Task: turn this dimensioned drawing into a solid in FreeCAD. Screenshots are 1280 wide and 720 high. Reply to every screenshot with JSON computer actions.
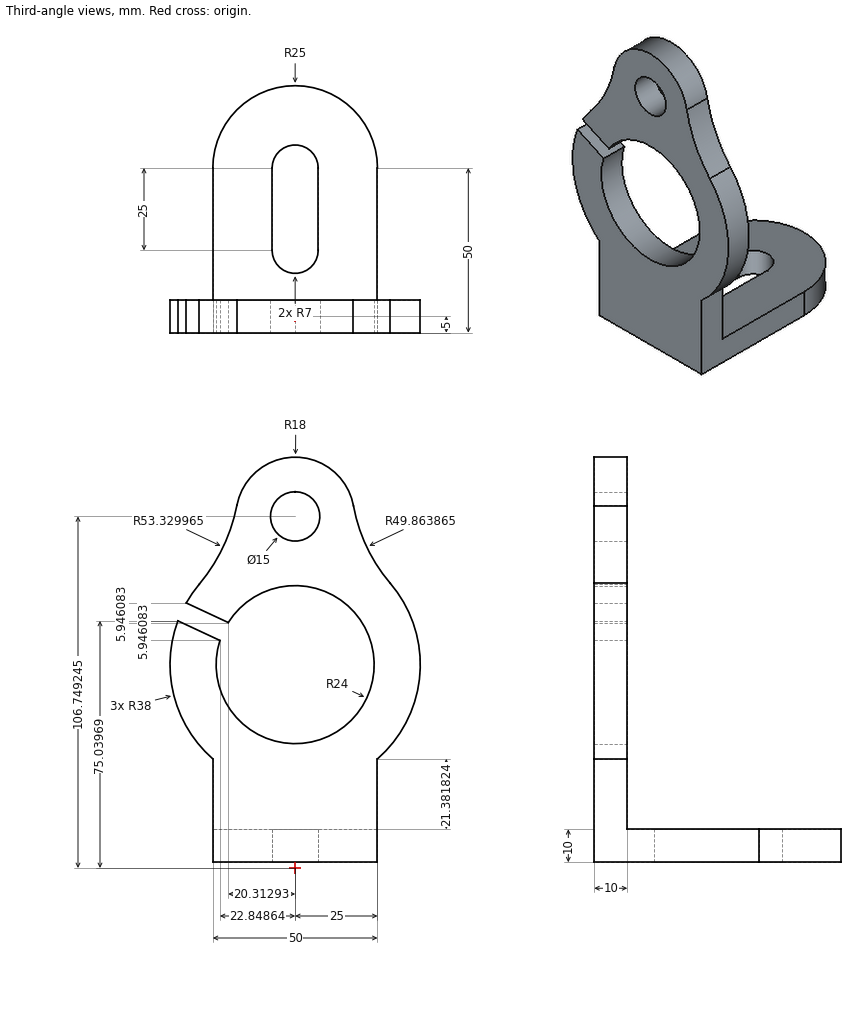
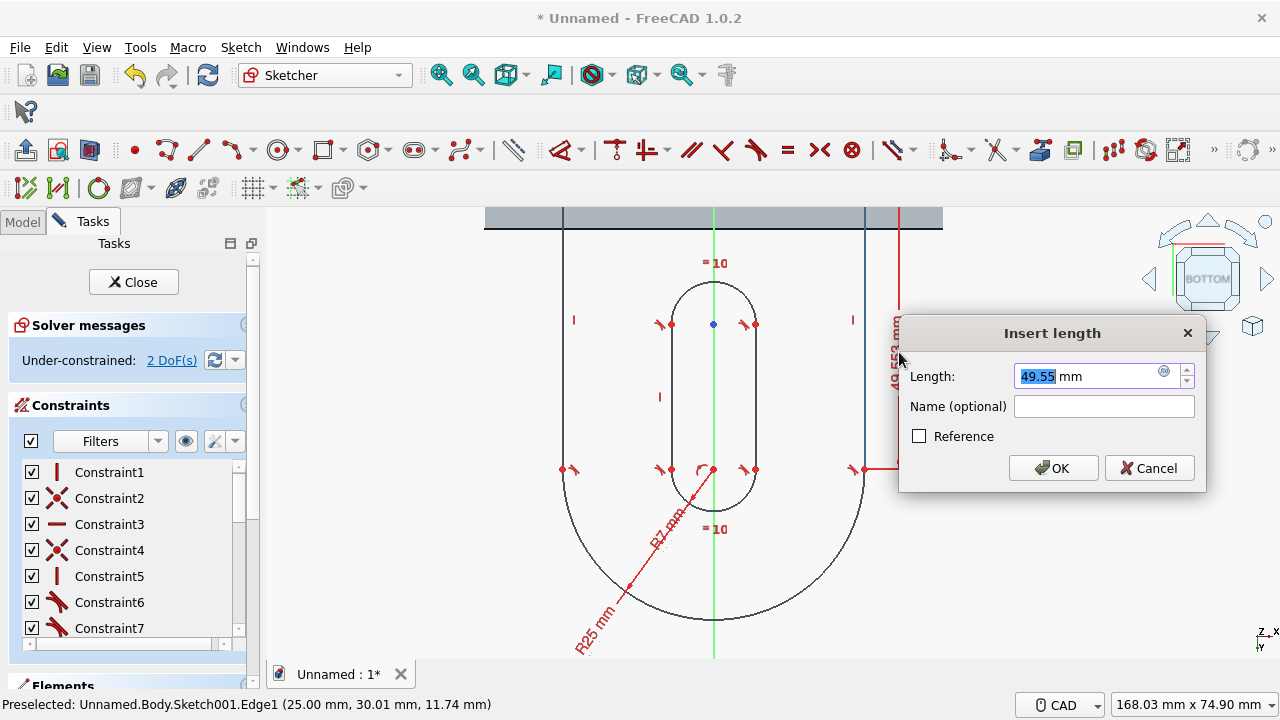
{"action": "type", "text": "50"}
{"action": "key", "text": "Return"}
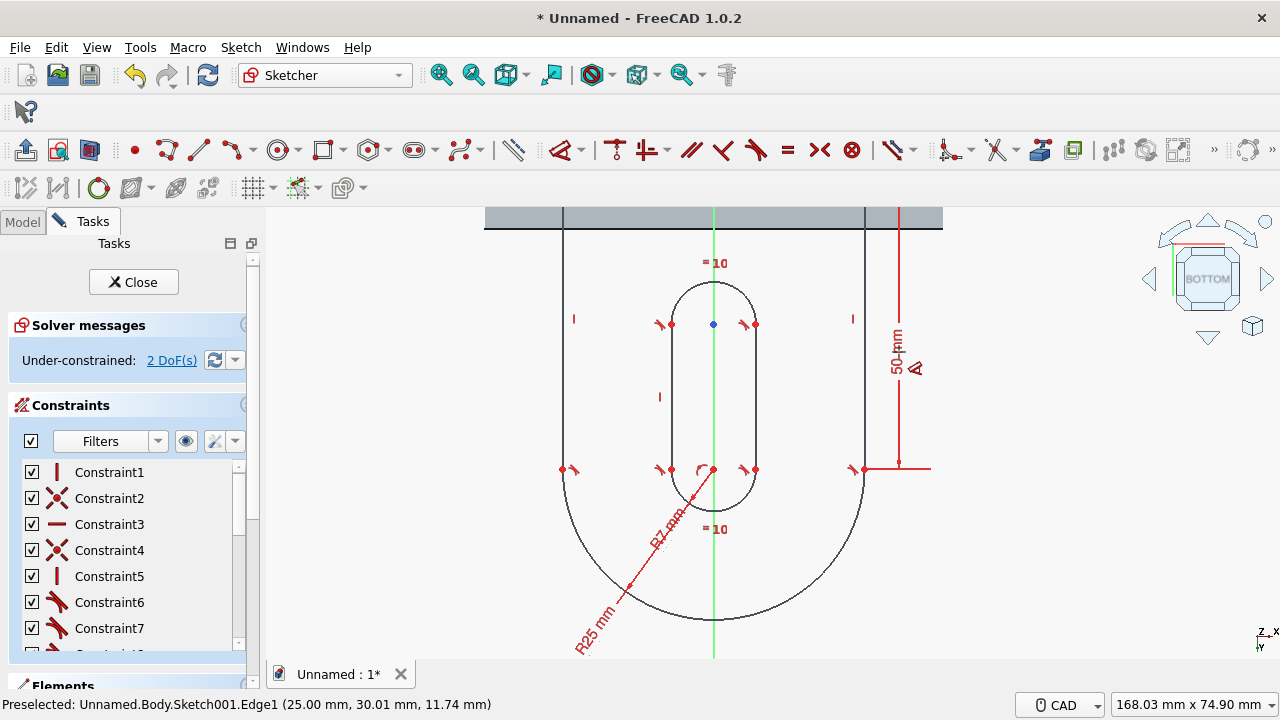
{"action": "left_click", "coordinate": [672, 426]}
{"action": "left_click", "coordinate": [638, 397]}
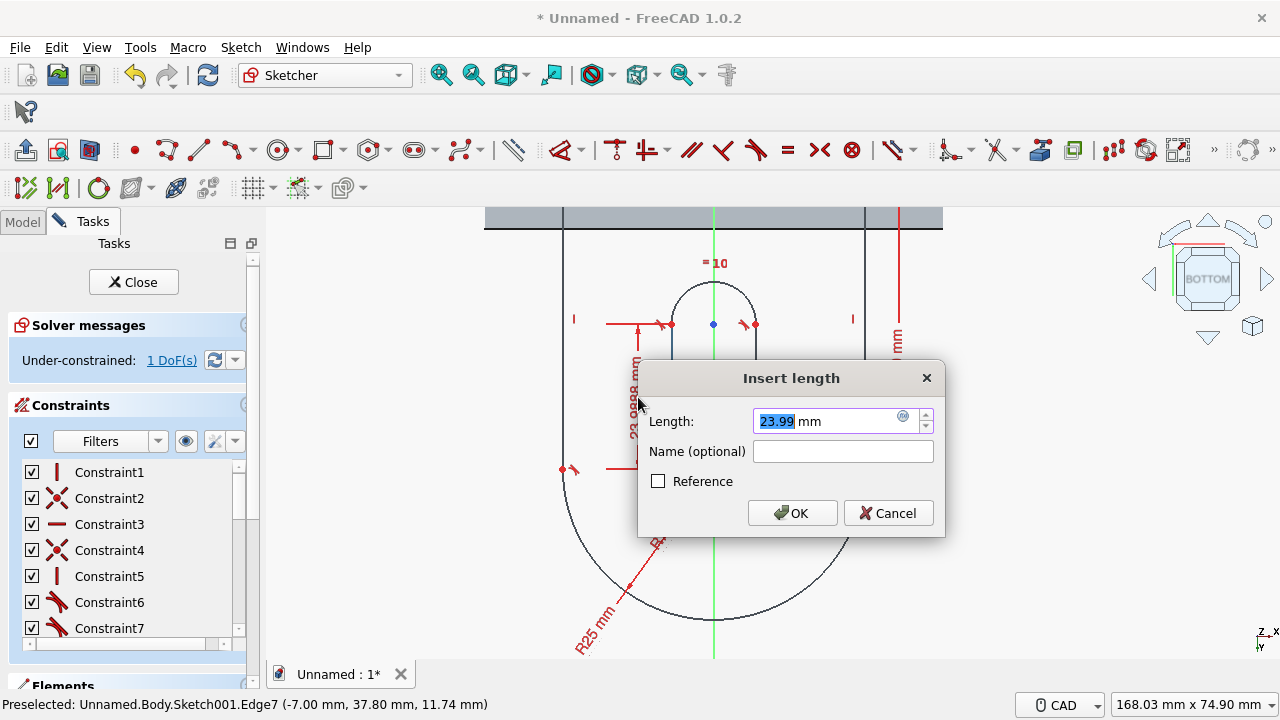
{"action": "type", "text": "25"}
{"action": "key", "text": "Return"}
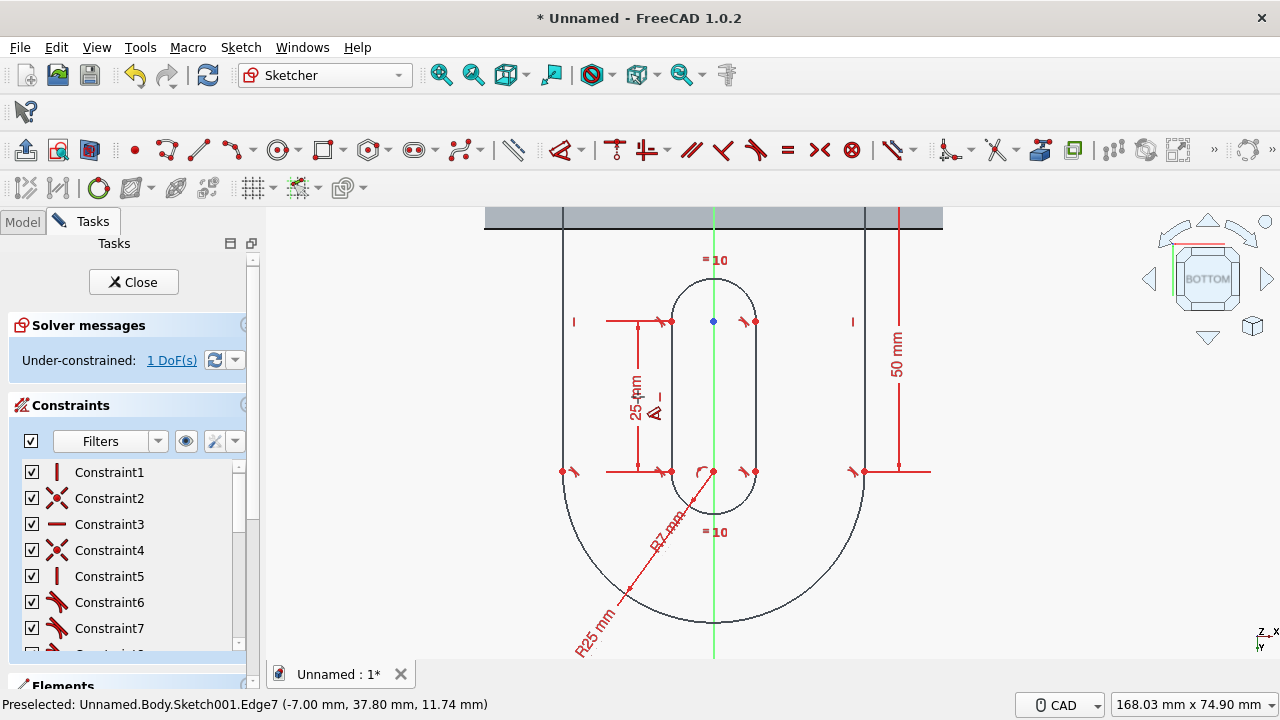
{"action": "scroll", "coordinate": [686, 510], "scroll_direction": "down", "scroll_amount": 2}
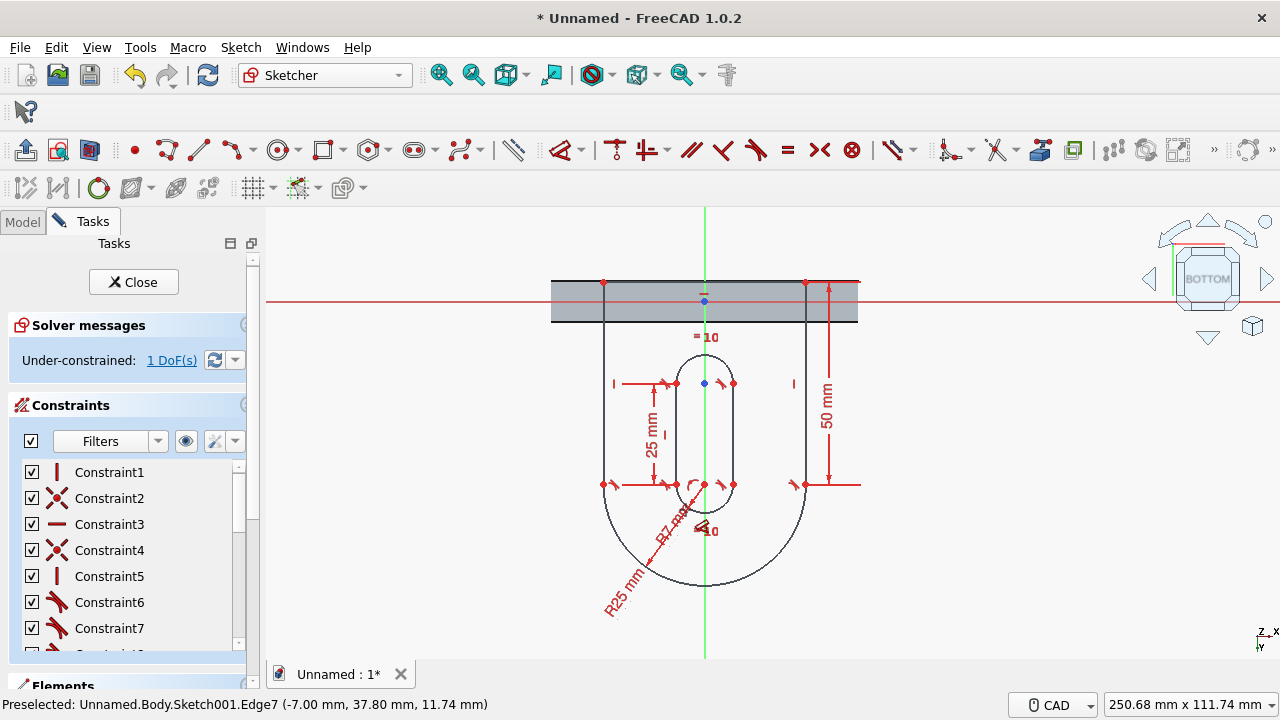
{"action": "scroll", "coordinate": [806, 282], "scroll_direction": "up", "scroll_amount": 4}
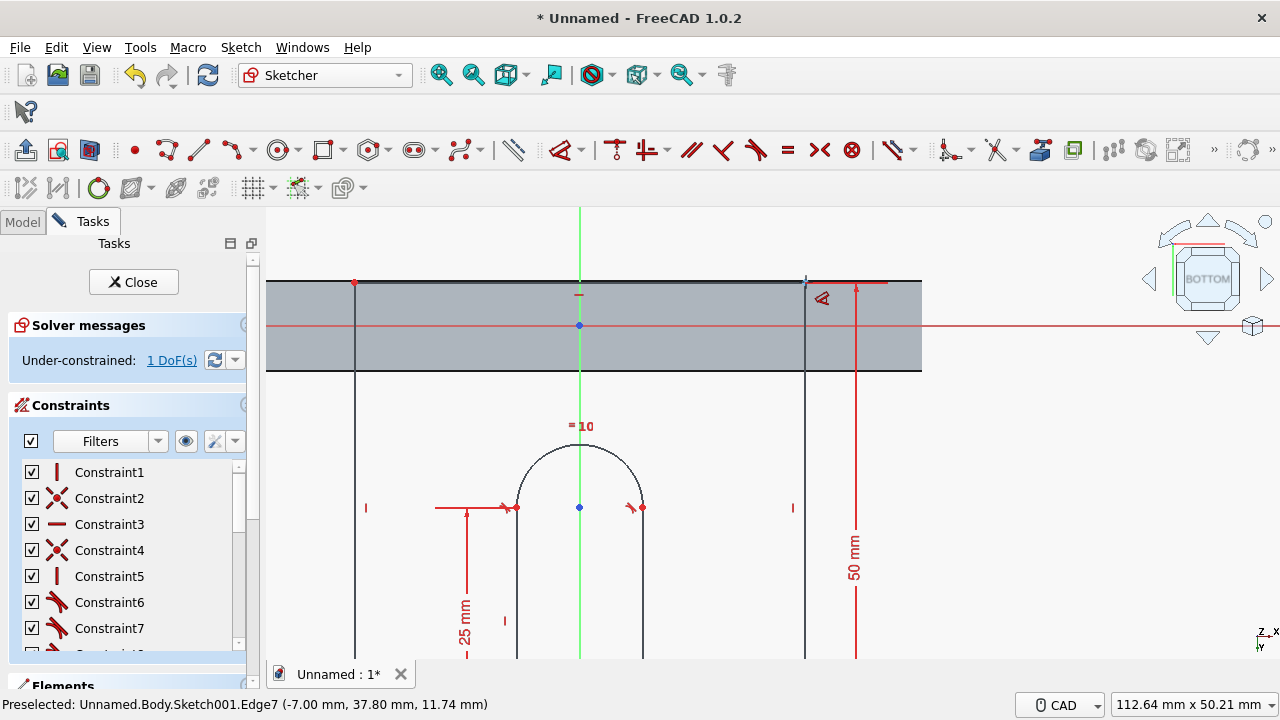
{"action": "left_click", "coordinate": [805, 283]}
{"action": "left_click", "coordinate": [839, 304]}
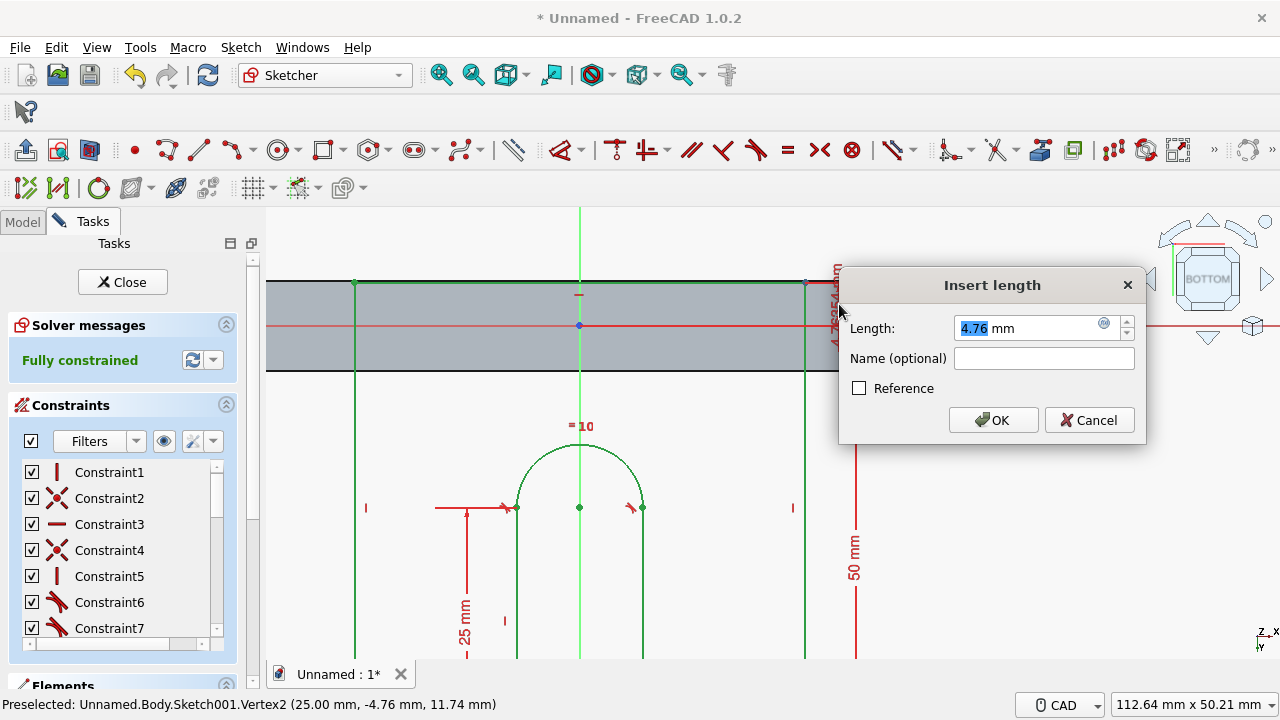
{"action": "type", "text": "5"}
{"action": "key", "text": "Return"}
{"action": "key", "text": "Escape"}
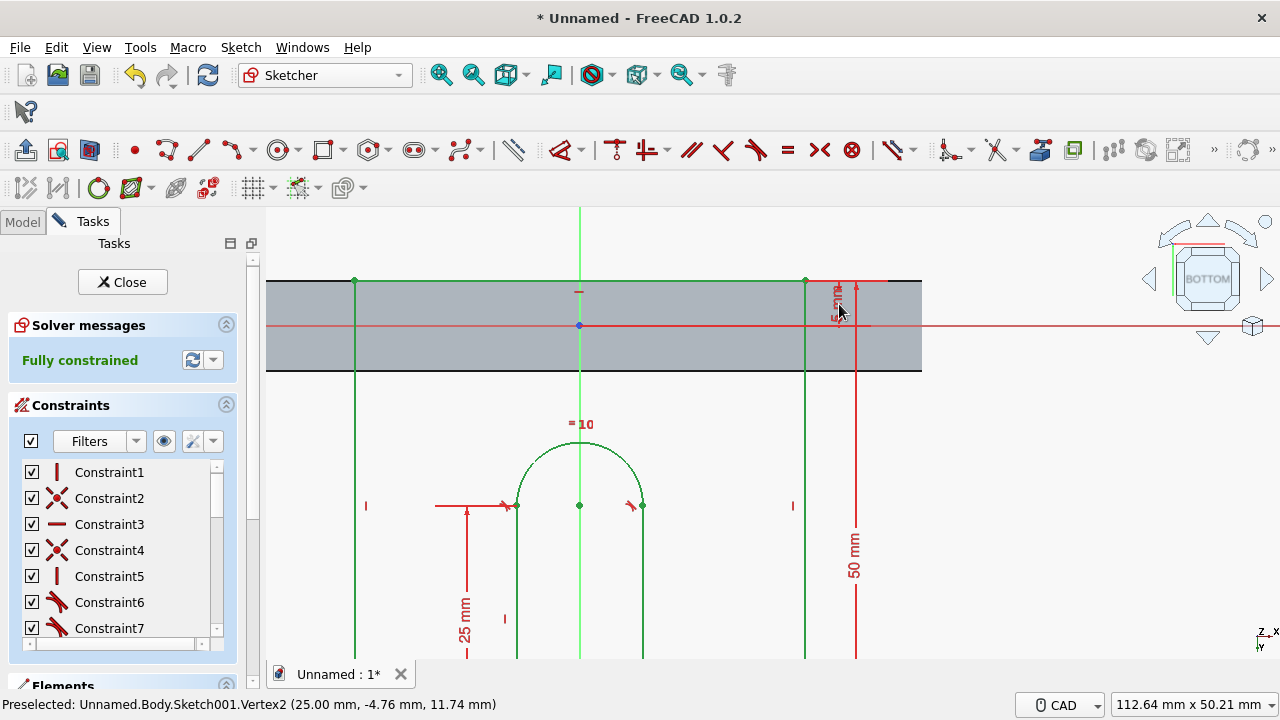
{"action": "left_click", "coordinate": [123, 282]}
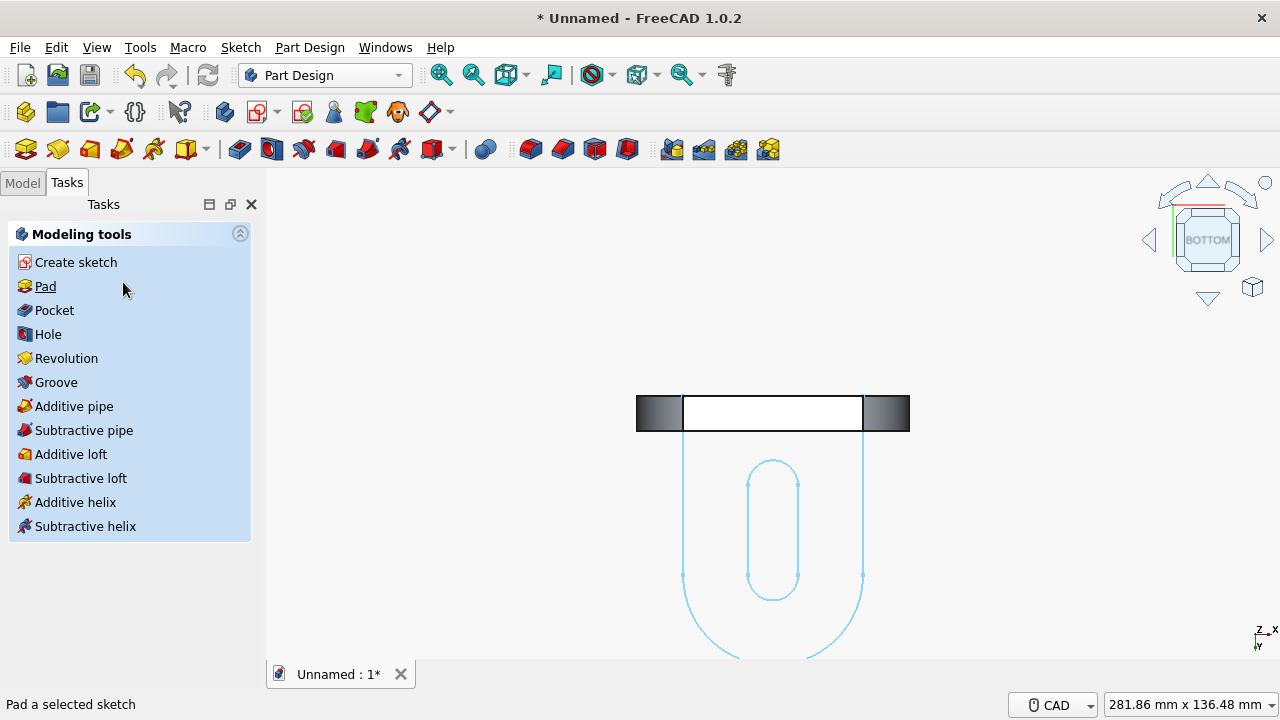
{"action": "left_click", "coordinate": [26, 150]}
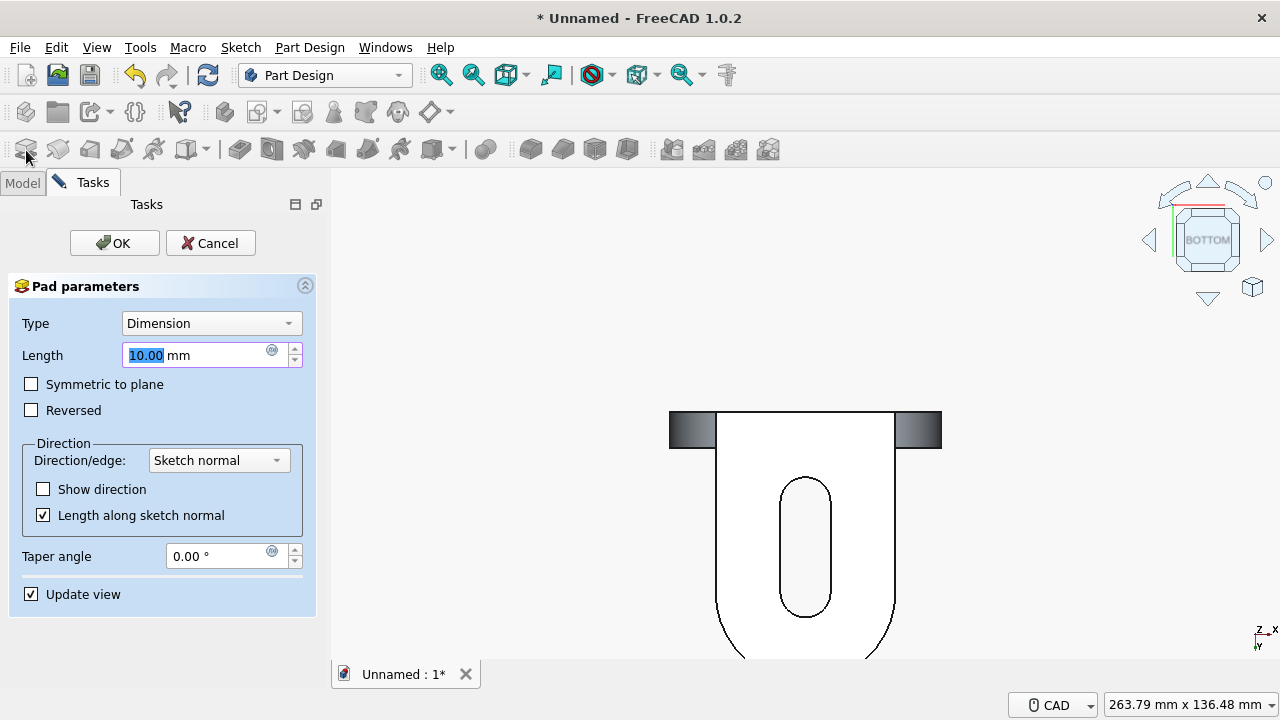
{"action": "type", "text": "10"}
{"action": "key", "text": "Tab"}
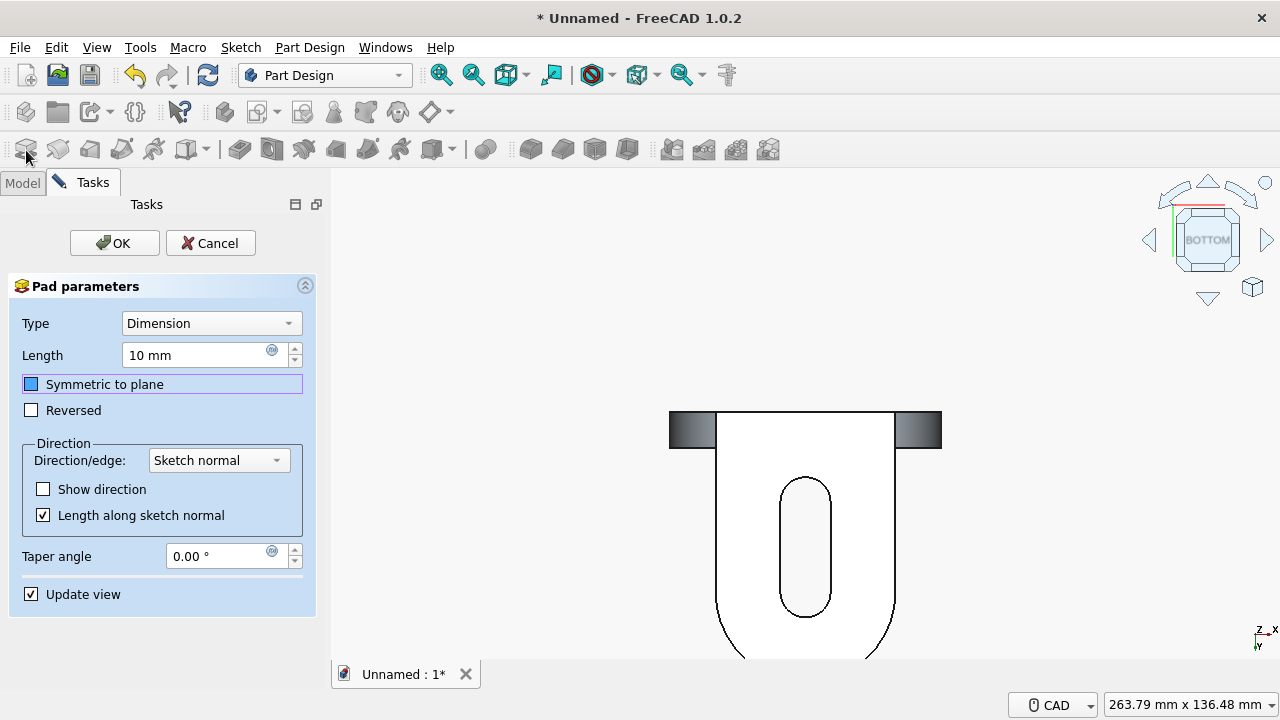
{"action": "left_click", "coordinate": [115, 243]}